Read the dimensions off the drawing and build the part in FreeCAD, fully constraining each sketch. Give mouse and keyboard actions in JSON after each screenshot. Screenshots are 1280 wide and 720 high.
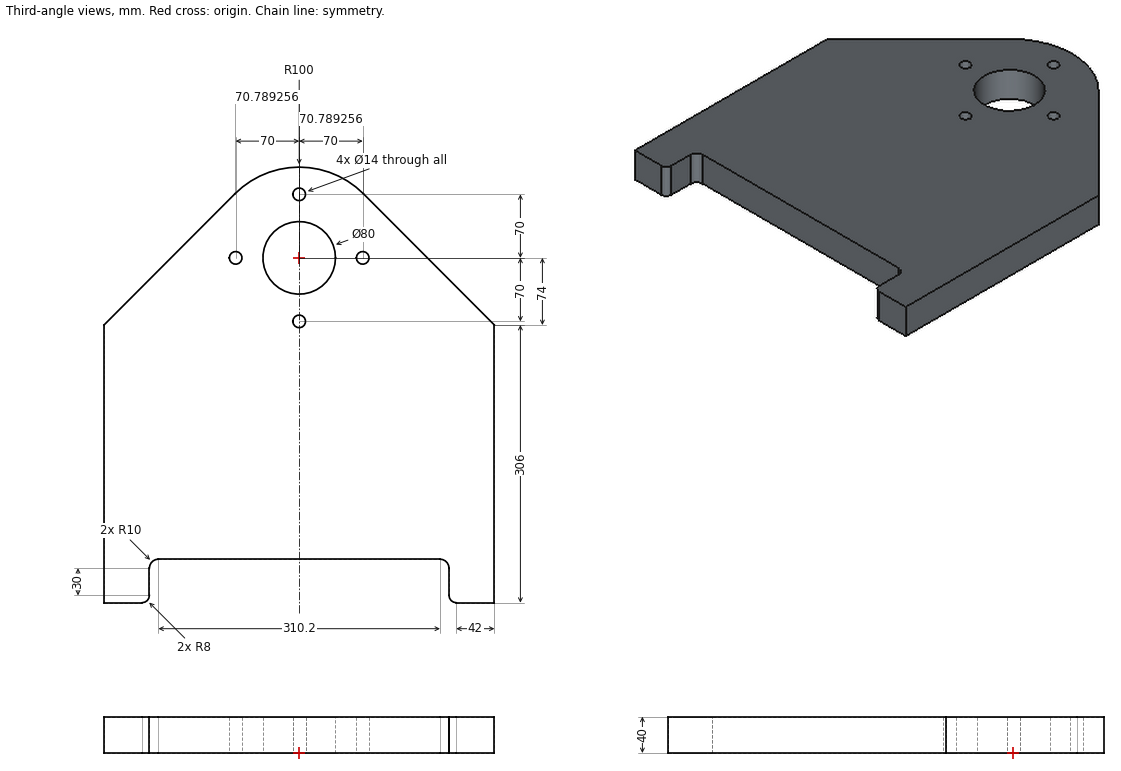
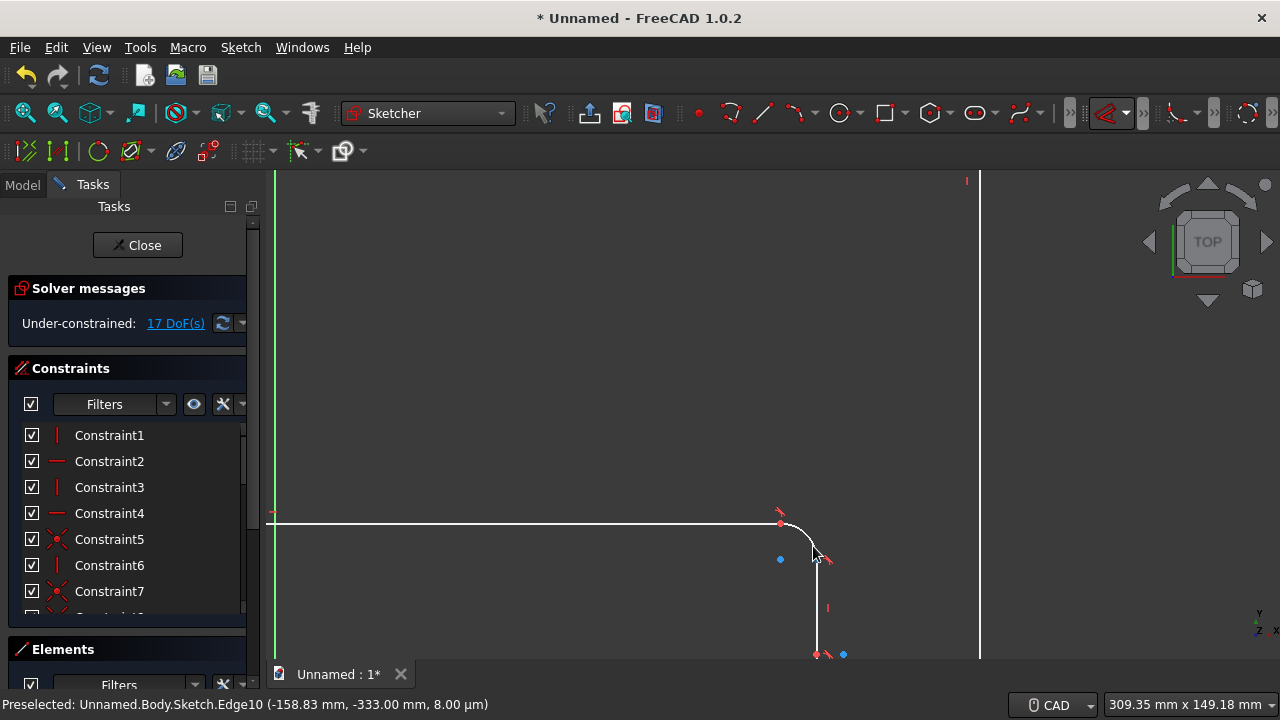
{"action": "left_click", "coordinate": [813, 543]}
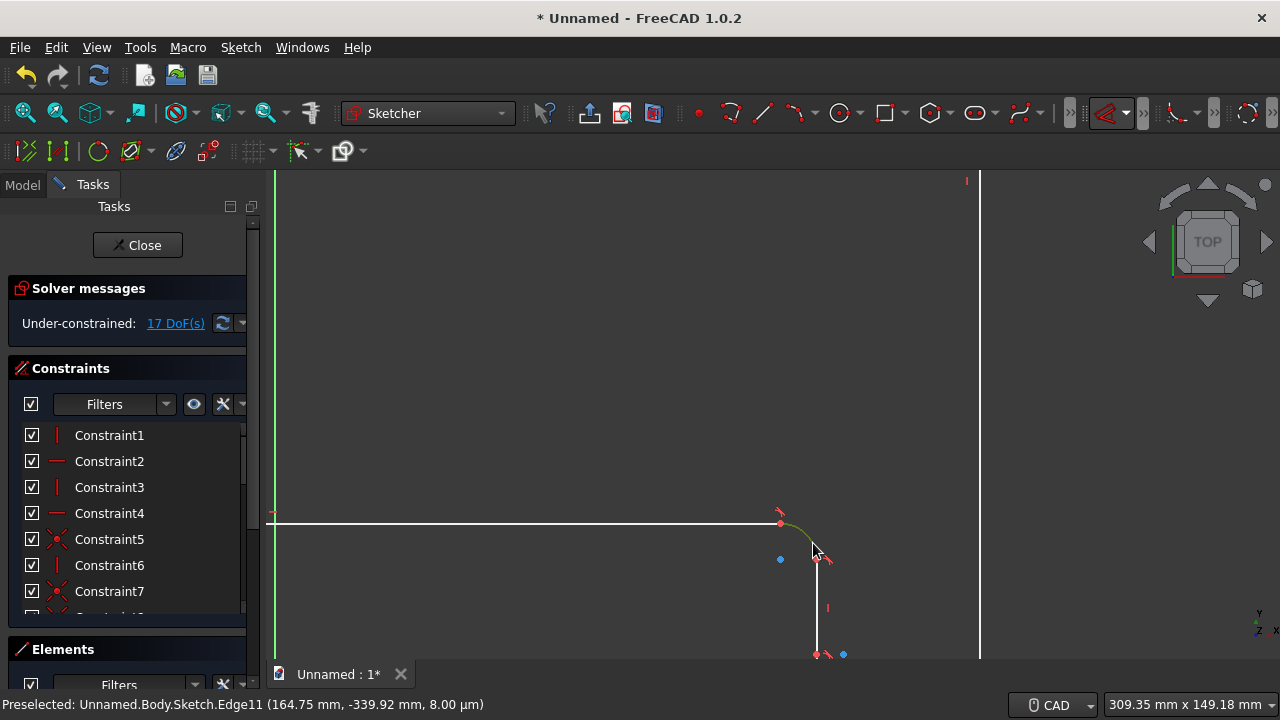
{"action": "key", "text": "e"}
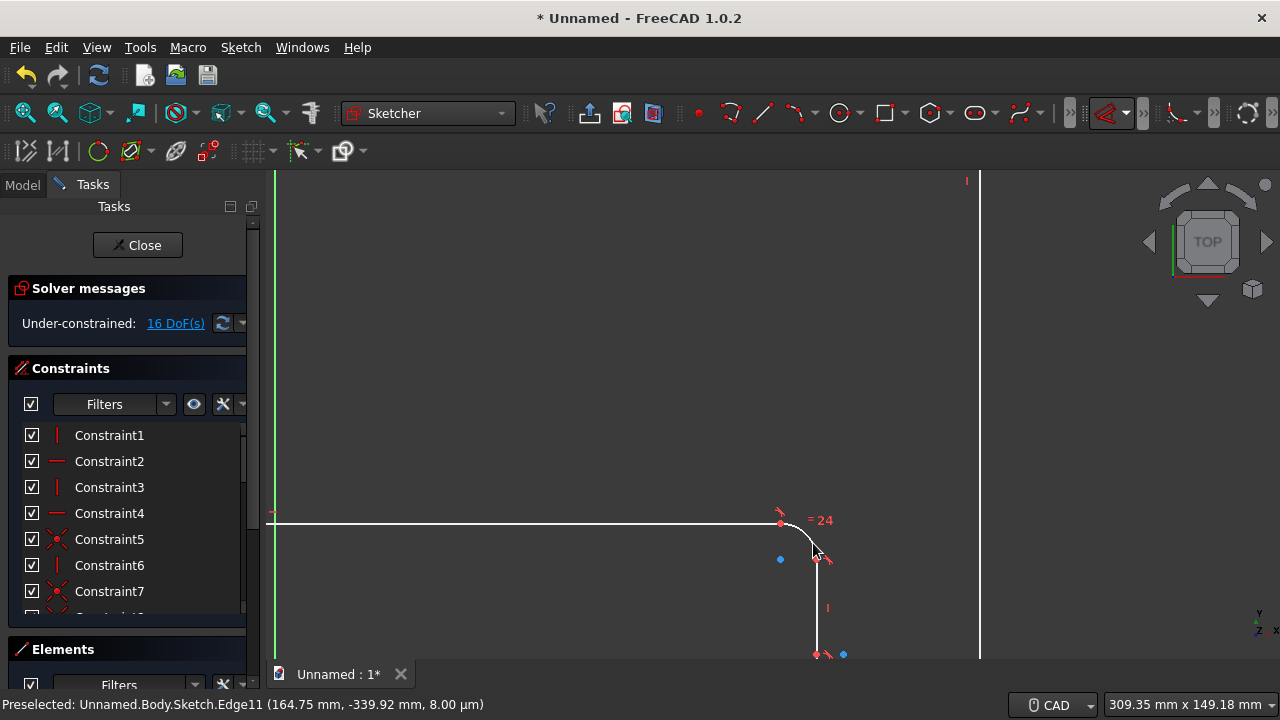
{"action": "scroll", "coordinate": [813, 546], "scroll_direction": "down", "scroll_amount": 8}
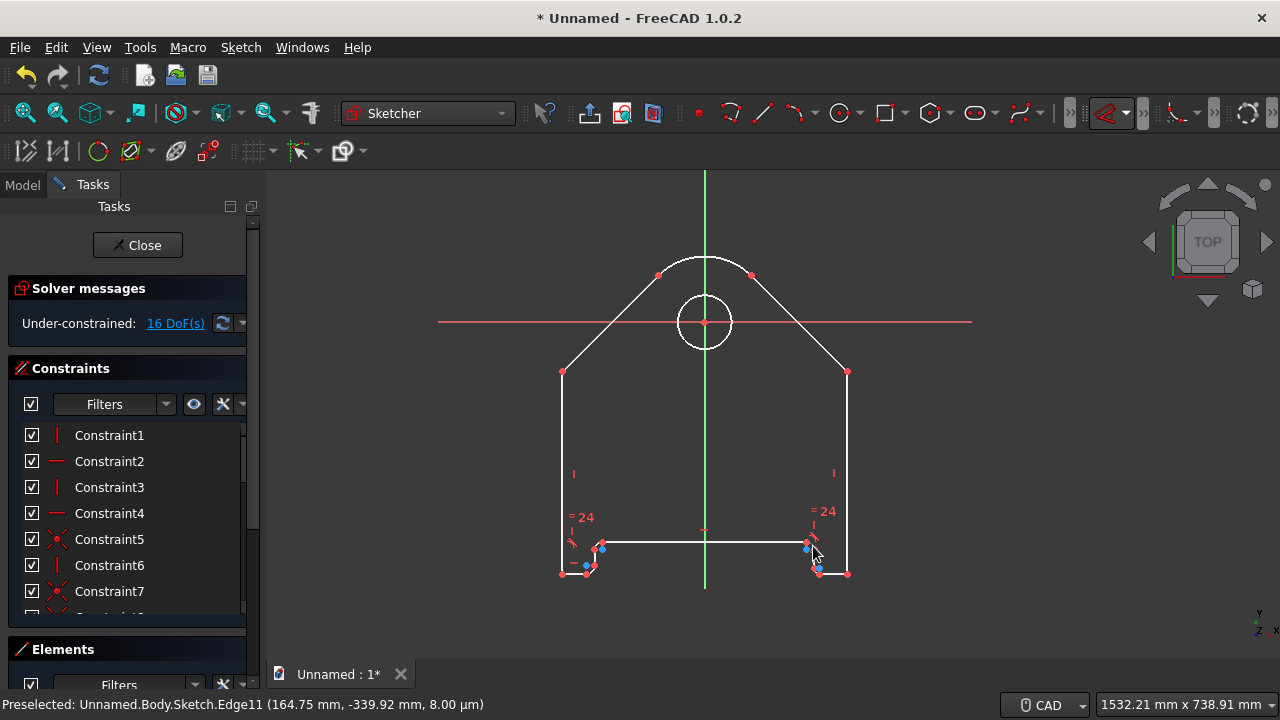
{"action": "scroll", "coordinate": [815, 571], "scroll_direction": "up", "scroll_amount": 9}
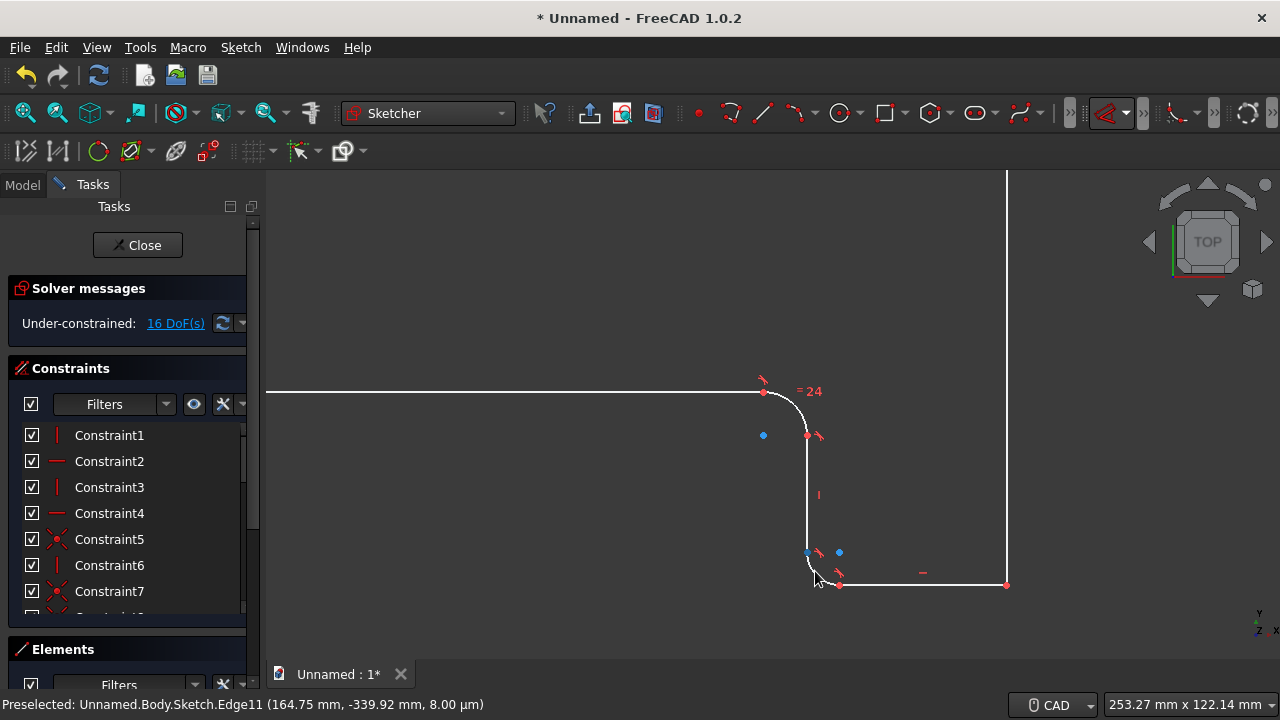
{"action": "left_click", "coordinate": [811, 567]}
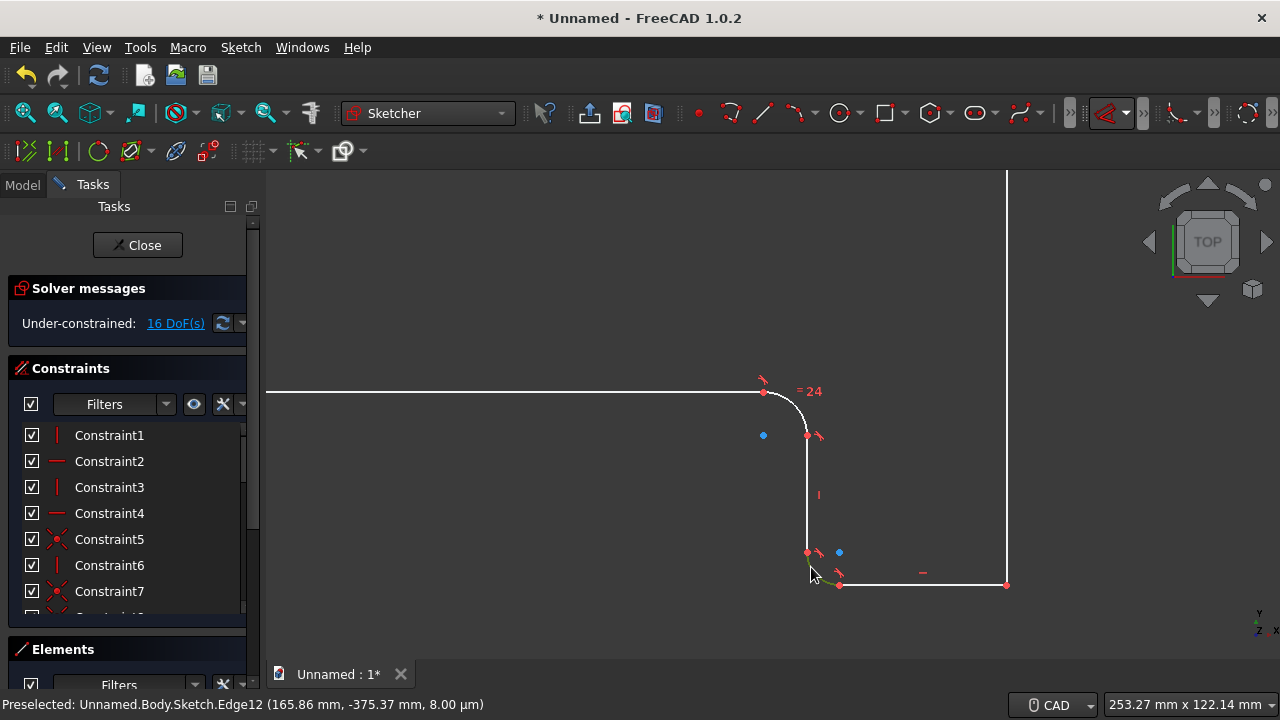
{"action": "scroll", "coordinate": [815, 571], "scroll_direction": "down", "scroll_amount": 9}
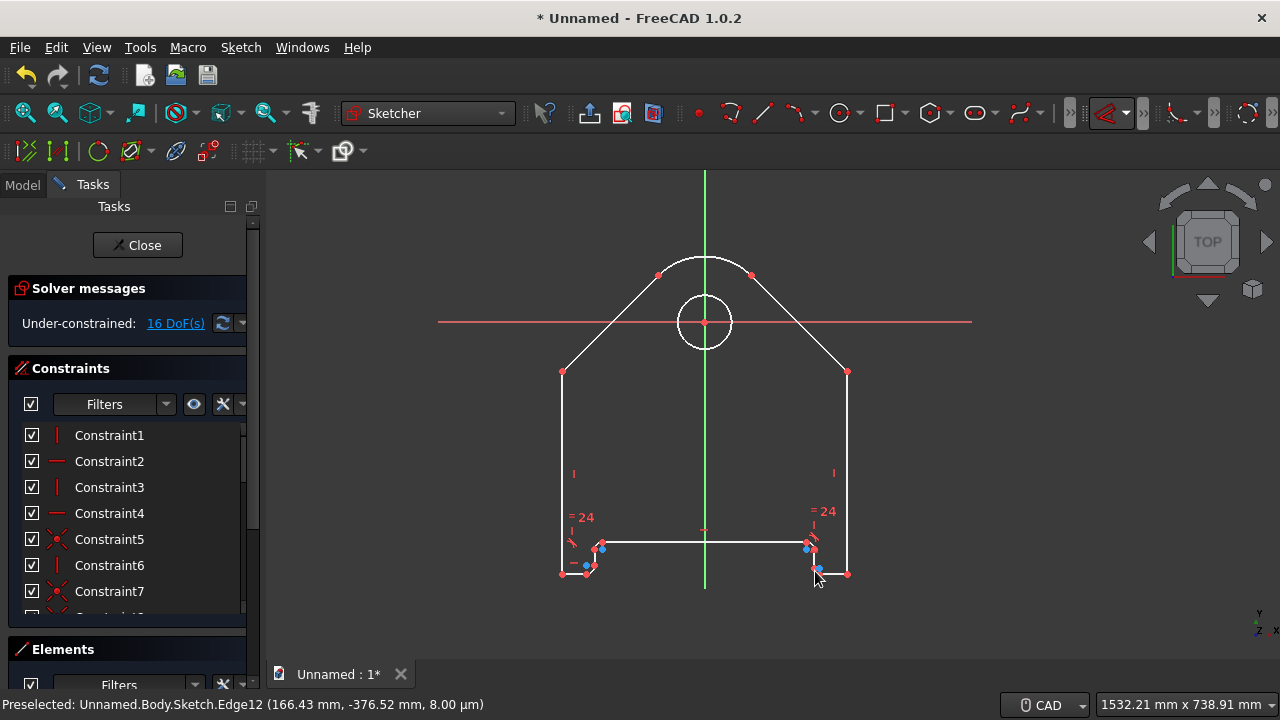
{"action": "scroll", "coordinate": [590, 573], "scroll_direction": "up", "scroll_amount": 7}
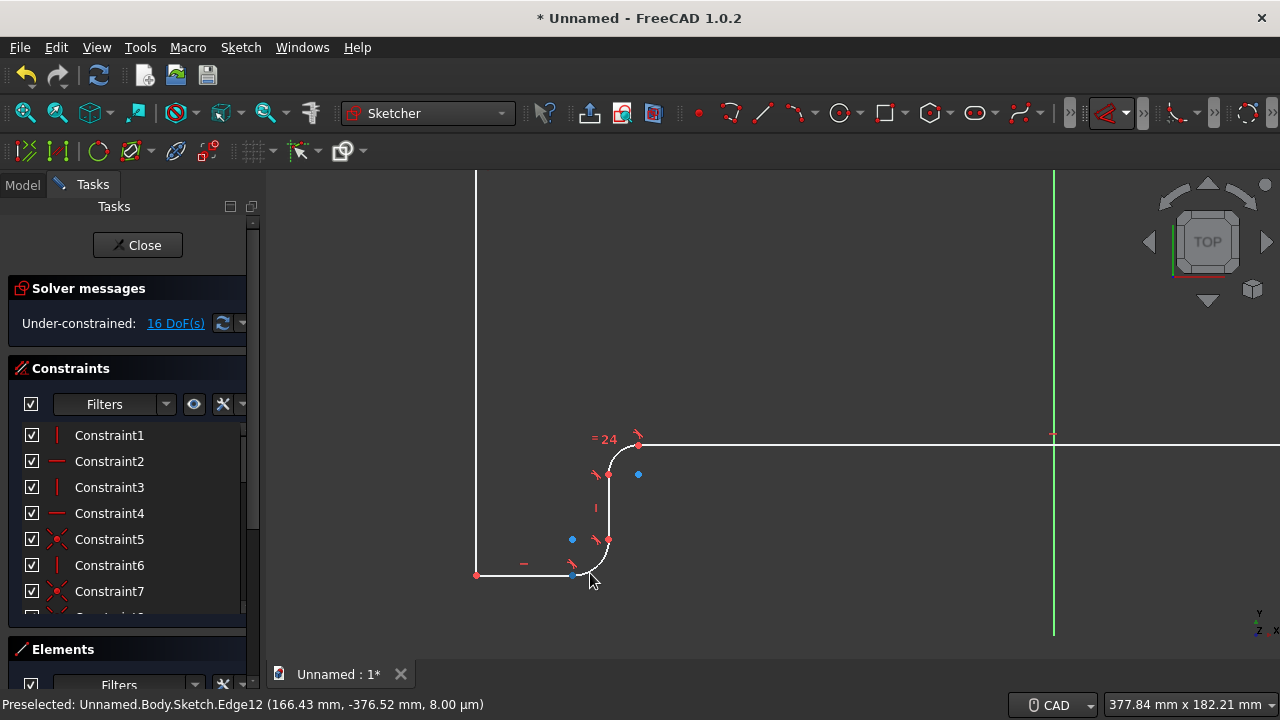
{"action": "left_click", "coordinate": [589, 572]}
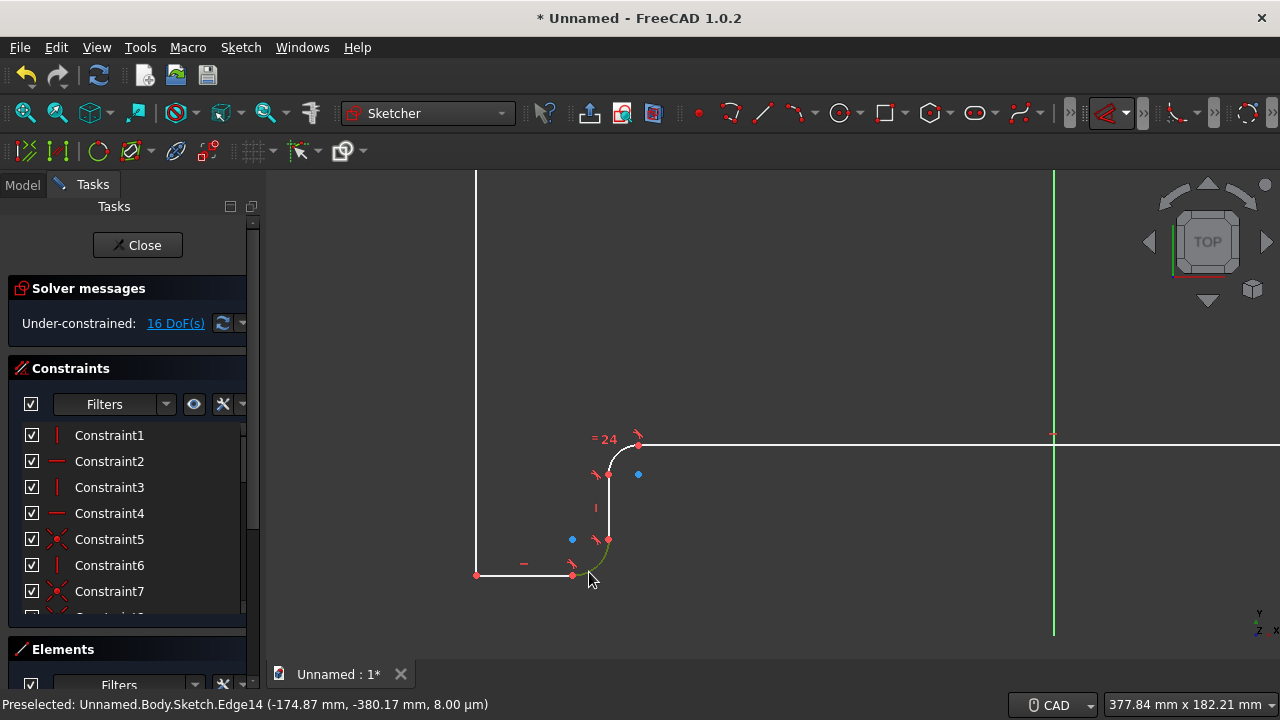
{"action": "key", "text": "e"}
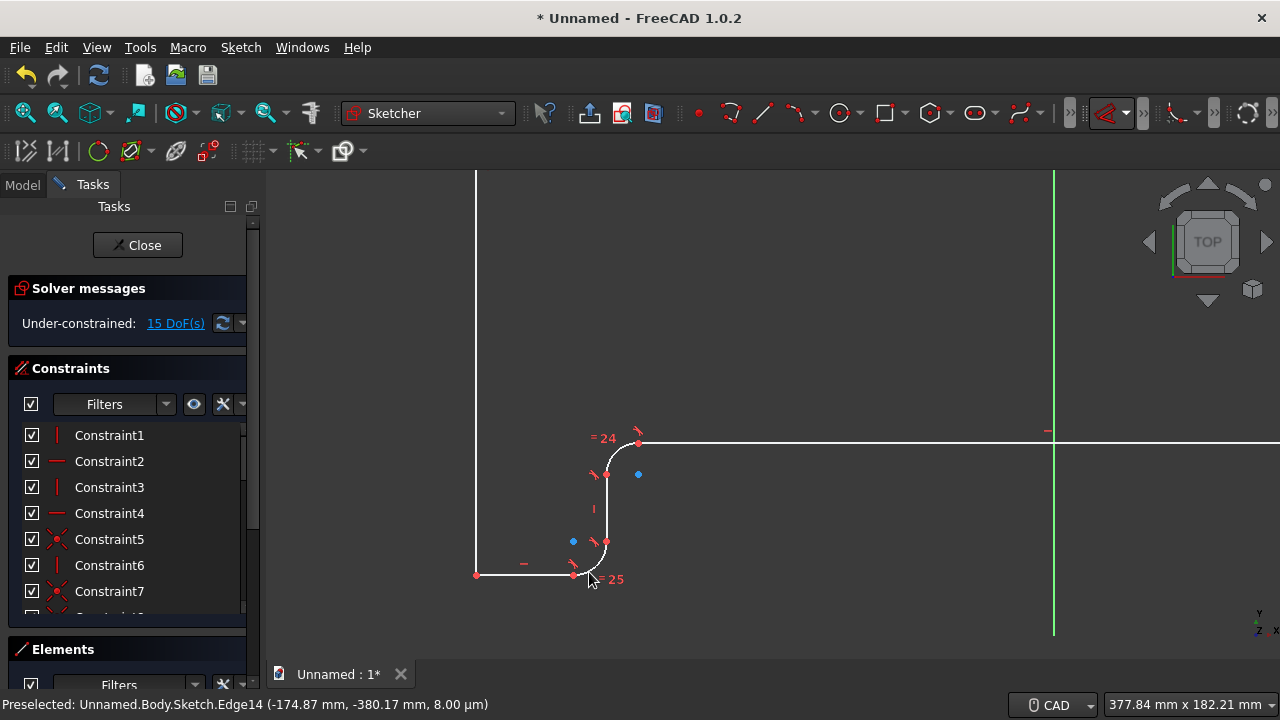
{"action": "scroll", "coordinate": [590, 573], "scroll_direction": "down", "scroll_amount": 7}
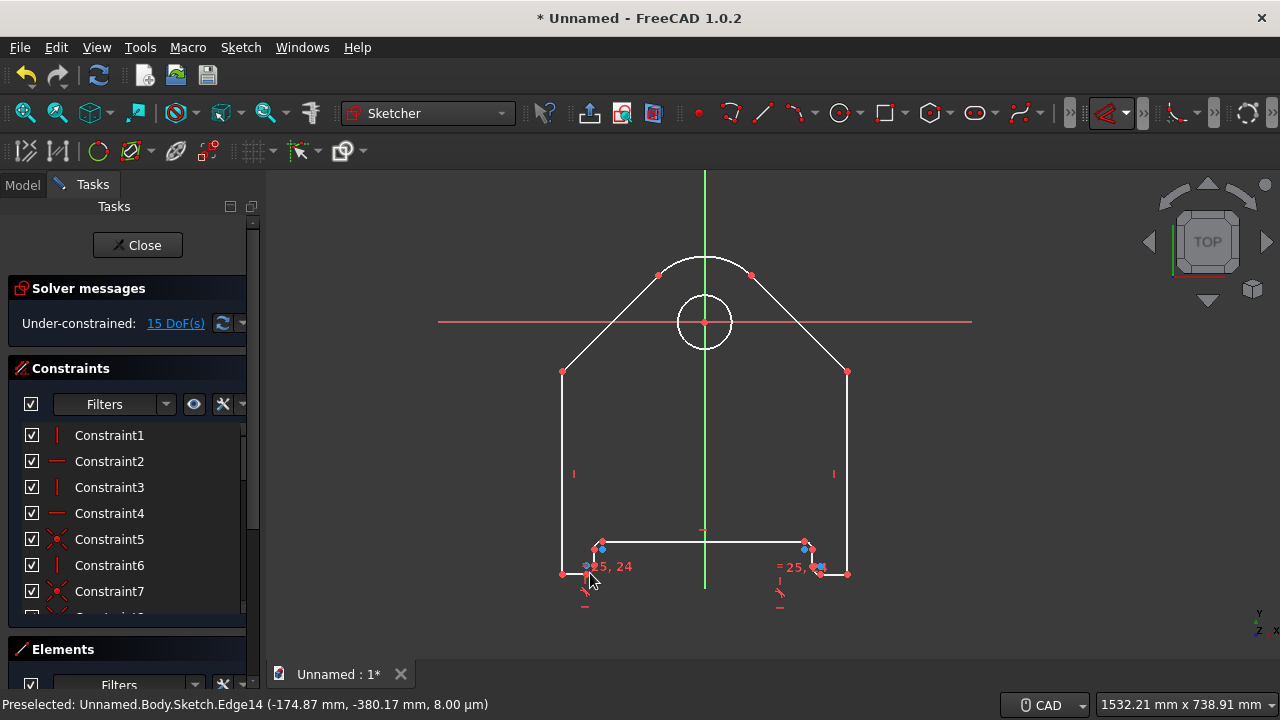
{"action": "scroll", "coordinate": [820, 567], "scroll_direction": "up", "scroll_amount": 2}